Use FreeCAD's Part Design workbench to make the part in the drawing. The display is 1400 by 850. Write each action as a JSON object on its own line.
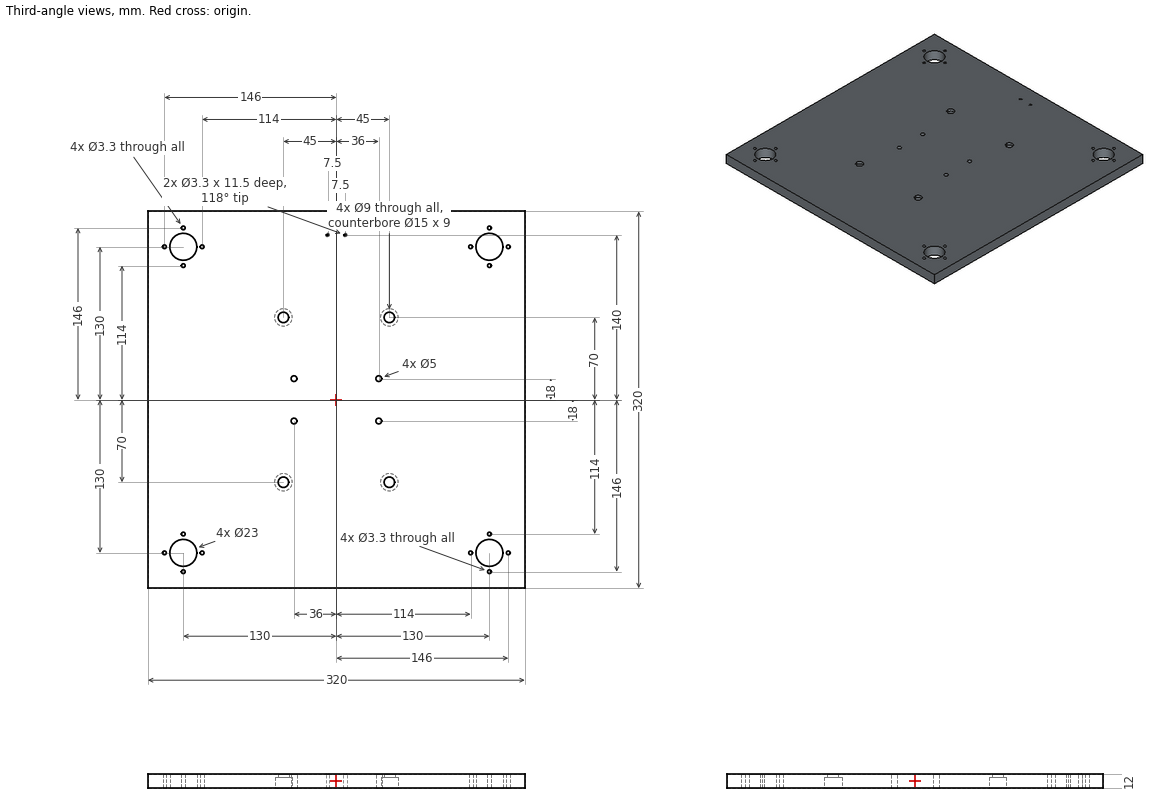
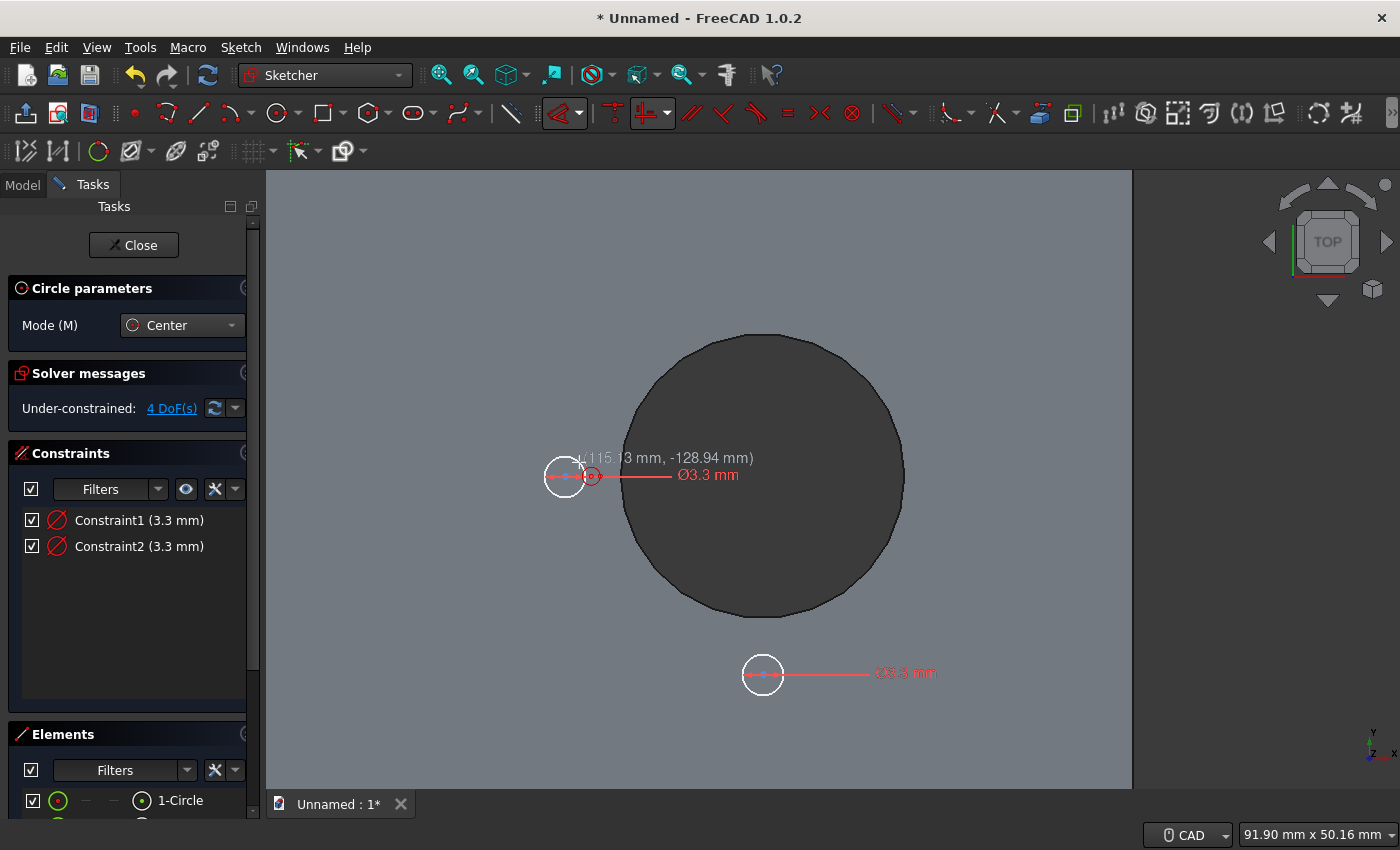
{"action": "left_click", "coordinate": [763, 279]}
{"action": "mouse_move", "coordinate": [777, 264]}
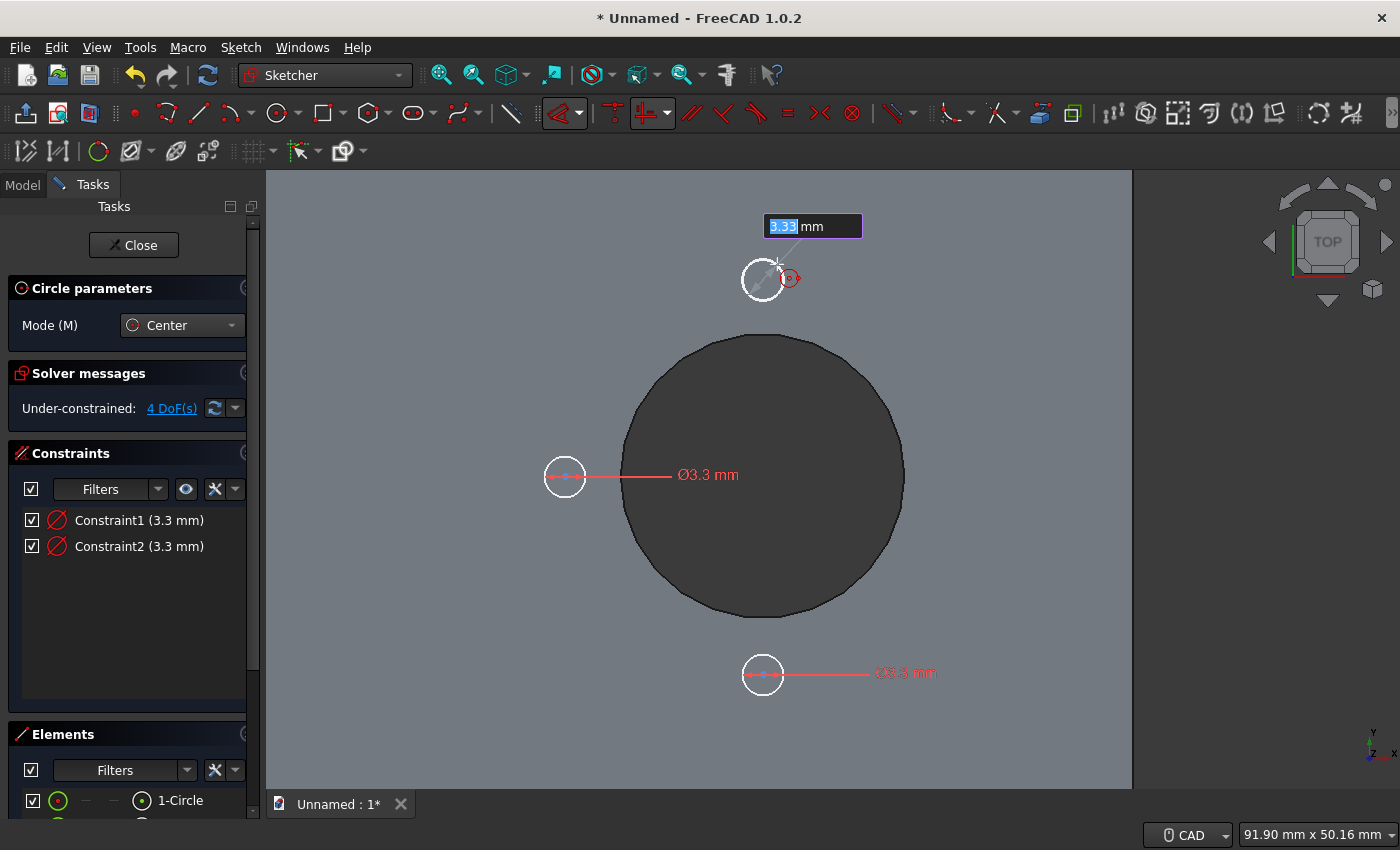
{"action": "type", "text": "3.3"}
{"action": "key", "text": "Return"}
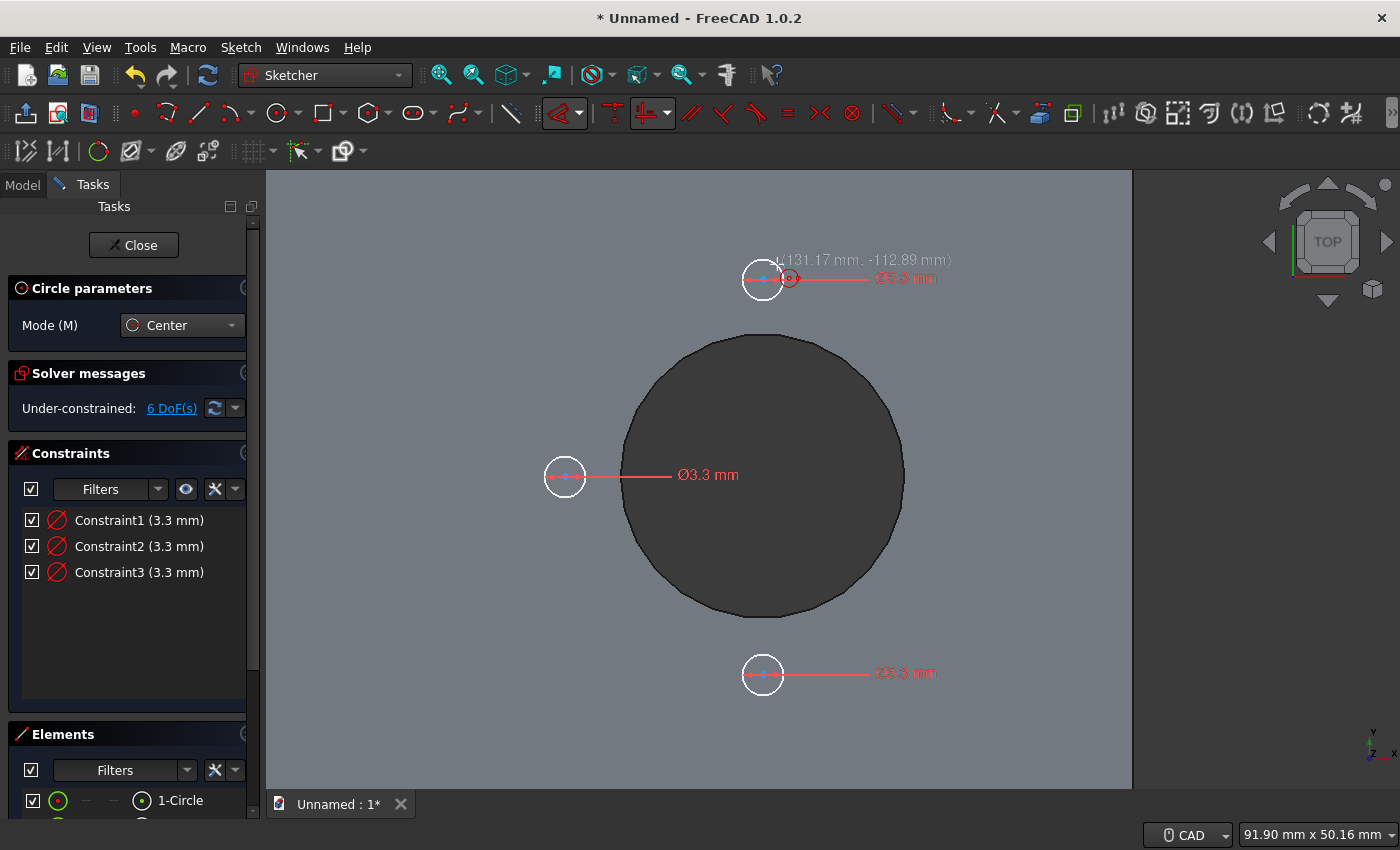
{"action": "left_click", "coordinate": [960, 476]}
{"action": "mouse_move", "coordinate": [974, 462]}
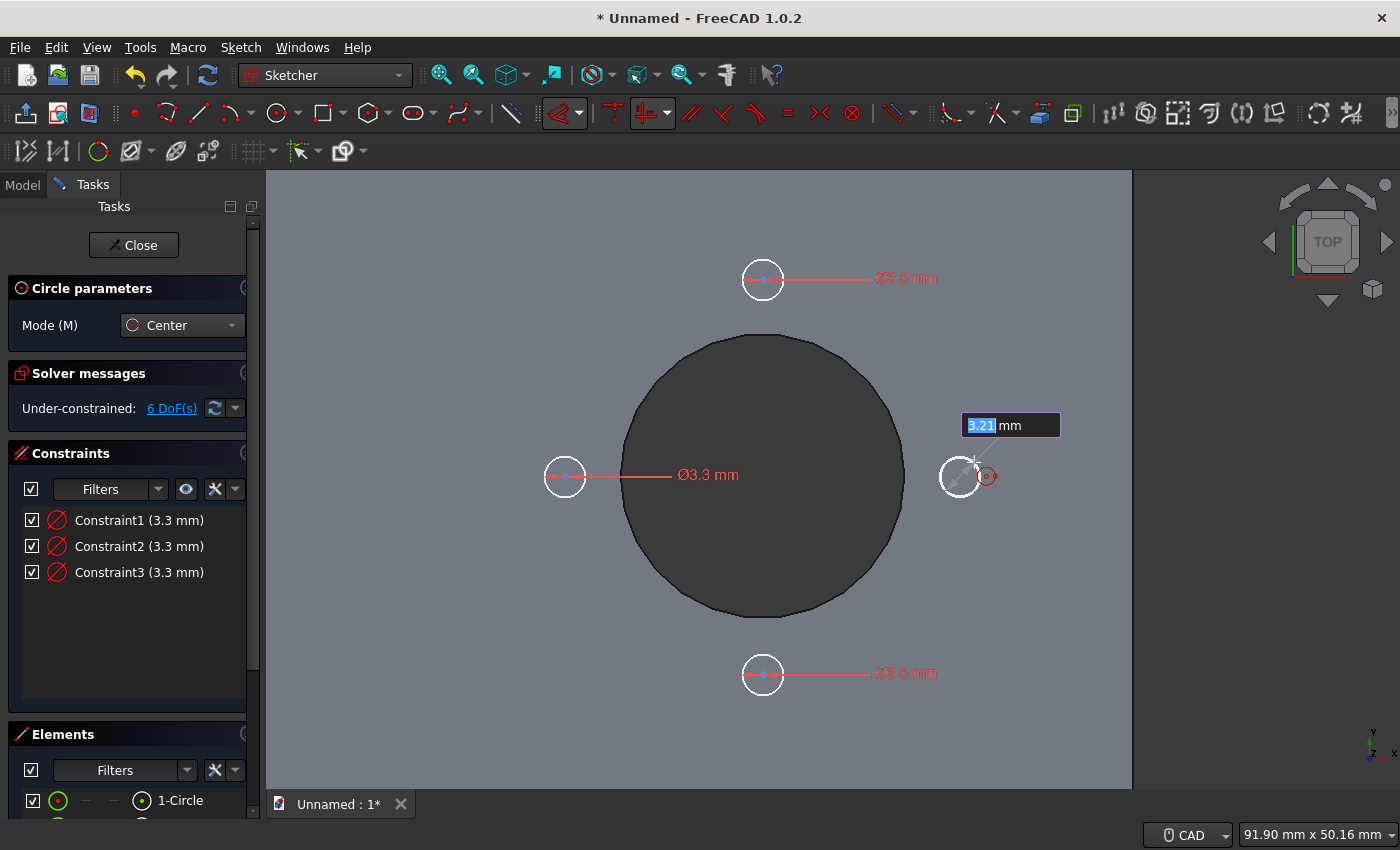
{"action": "type", "text": "3.3"}
{"action": "key", "text": "Return"}
{"action": "key", "text": "Escape"}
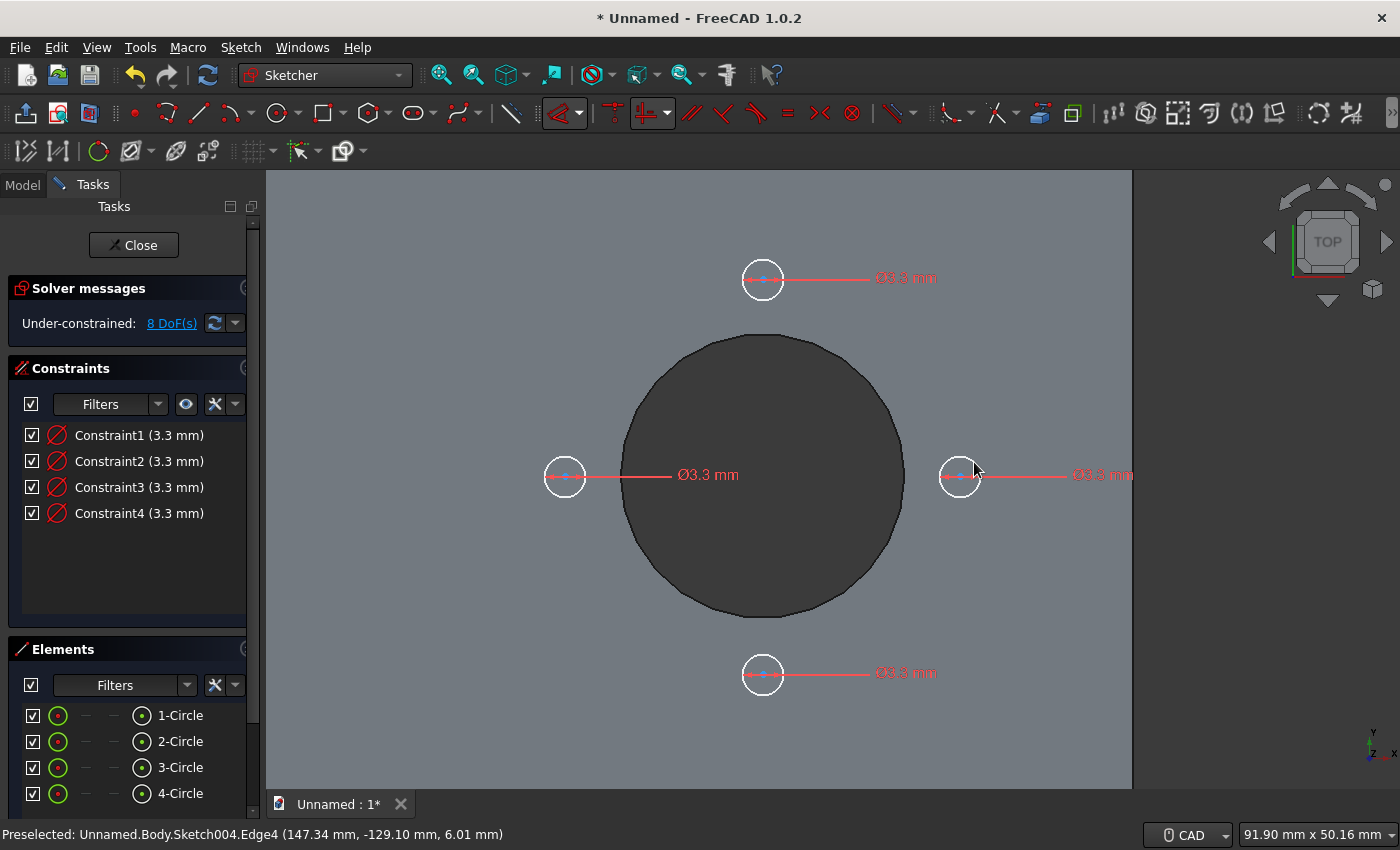
{"action": "left_click", "coordinate": [763, 675]}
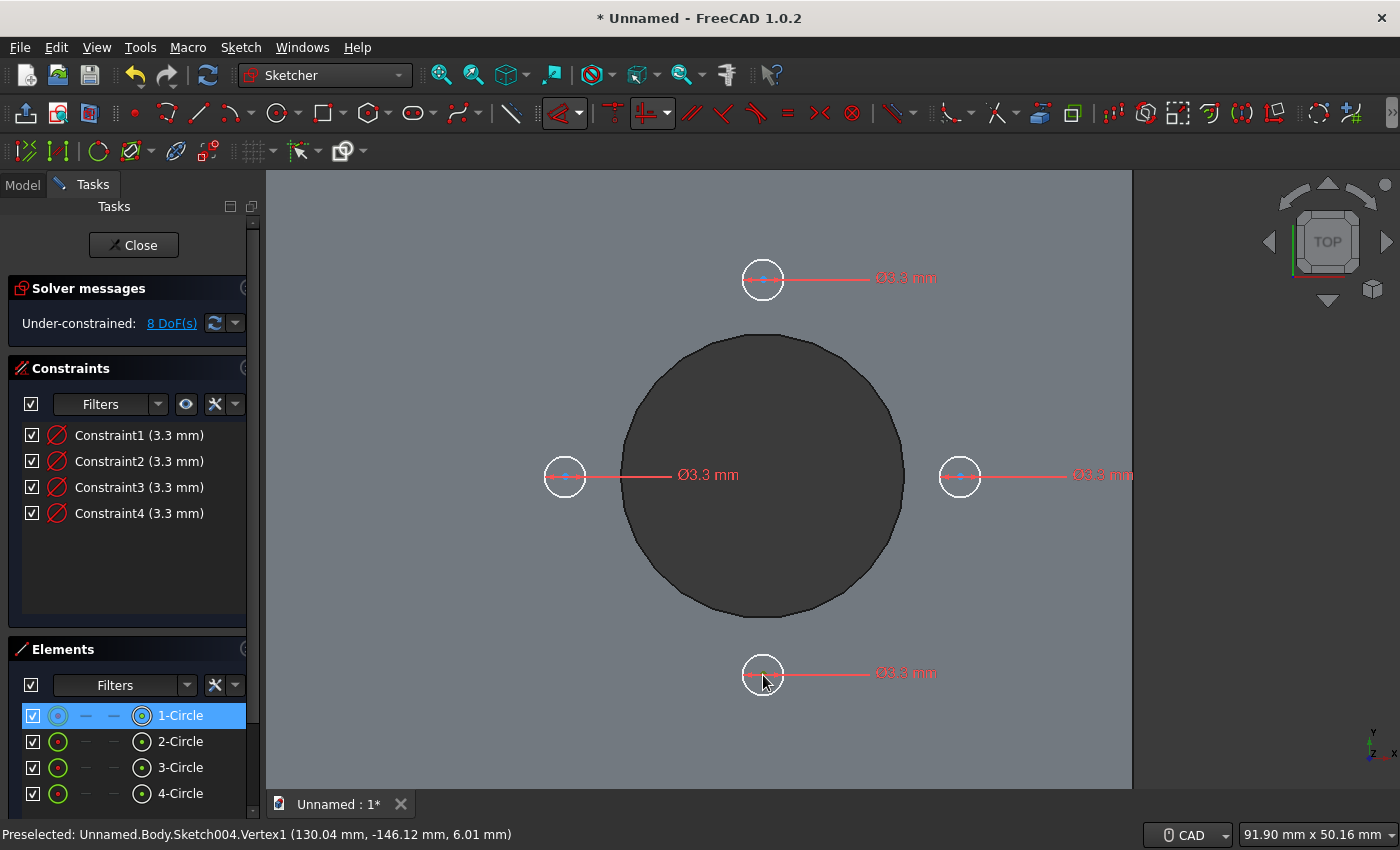
{"action": "left_click", "coordinate": [763, 280]}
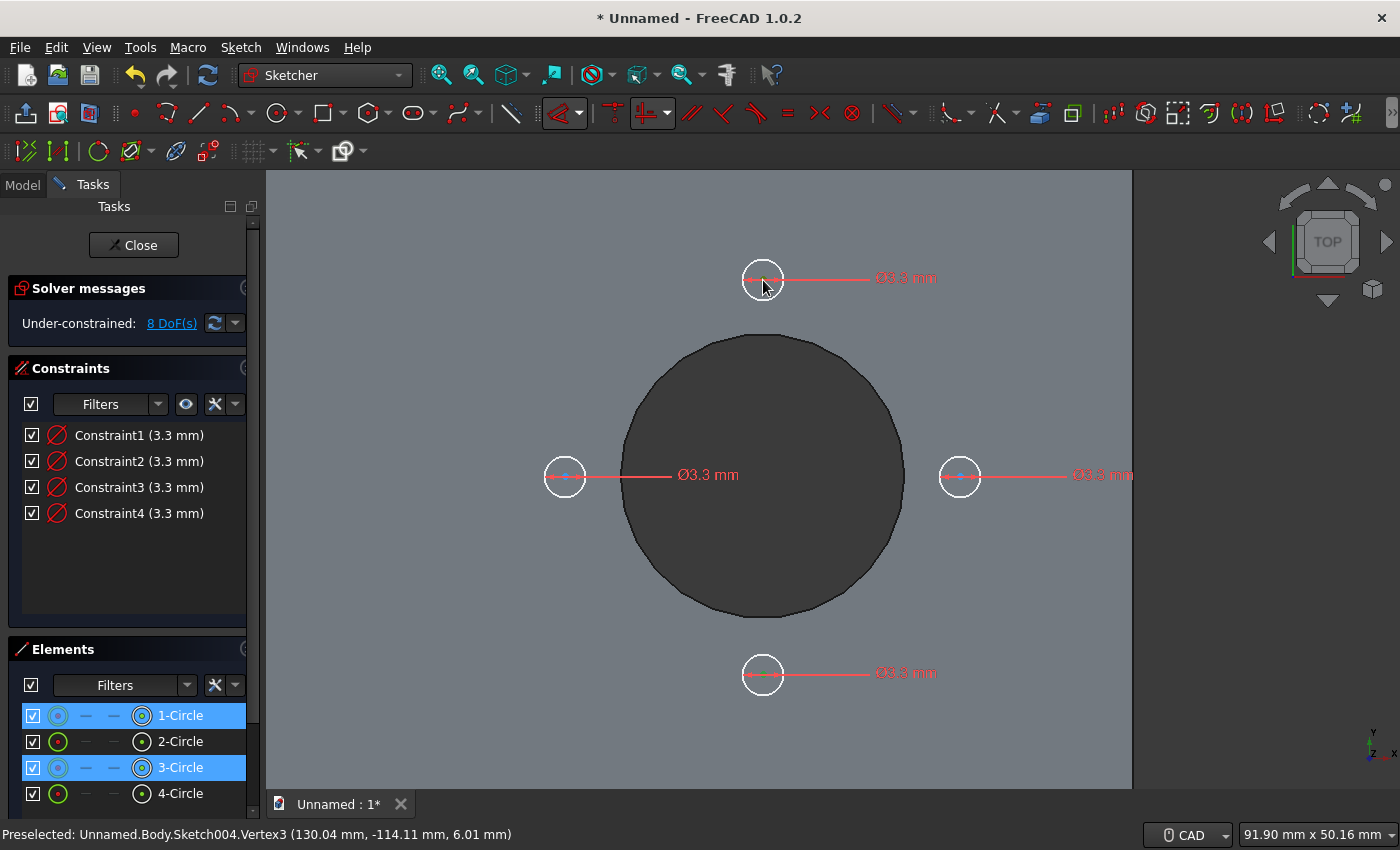
{"action": "left_click", "coordinate": [670, 114]}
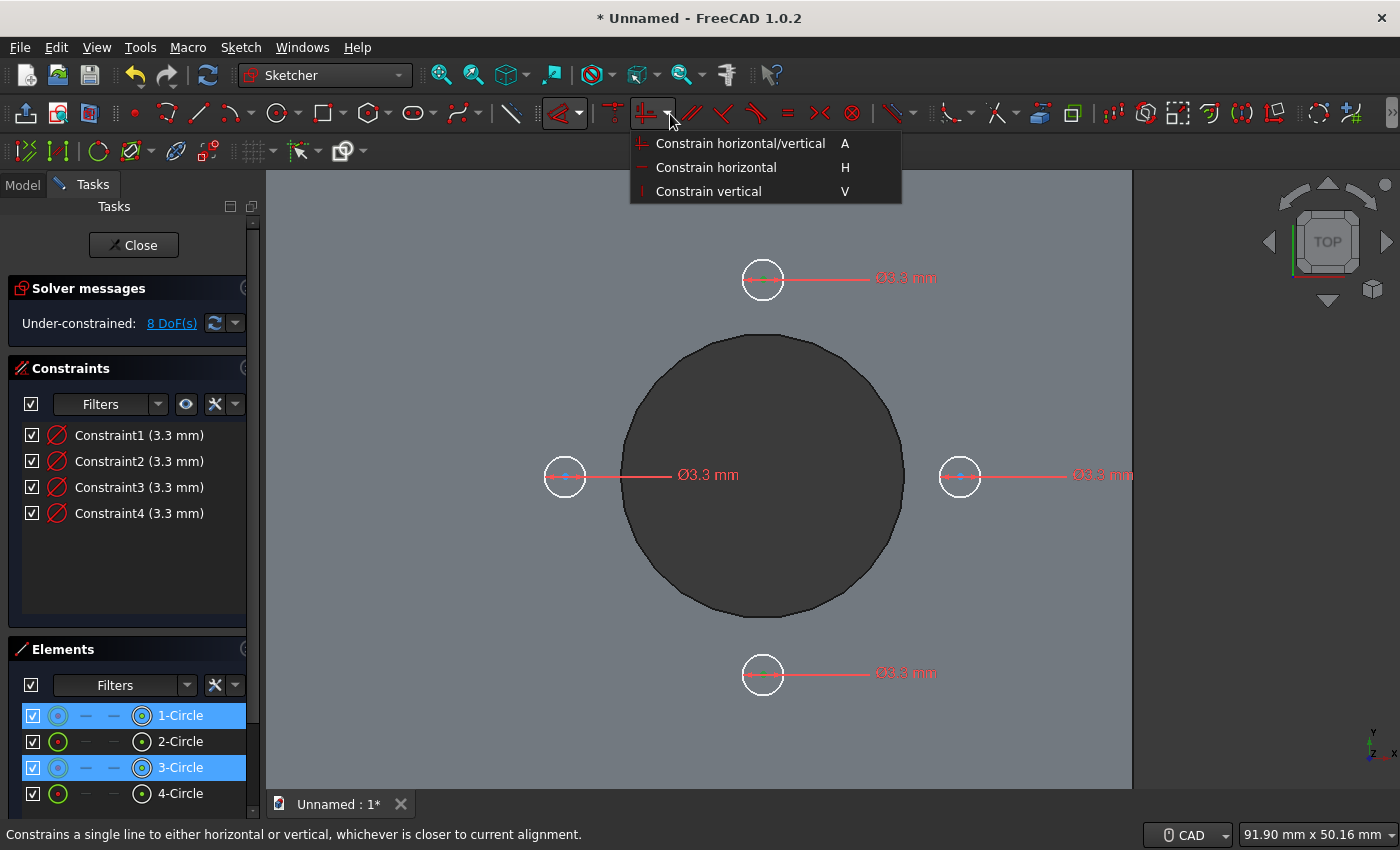
{"action": "left_click", "coordinate": [766, 191]}